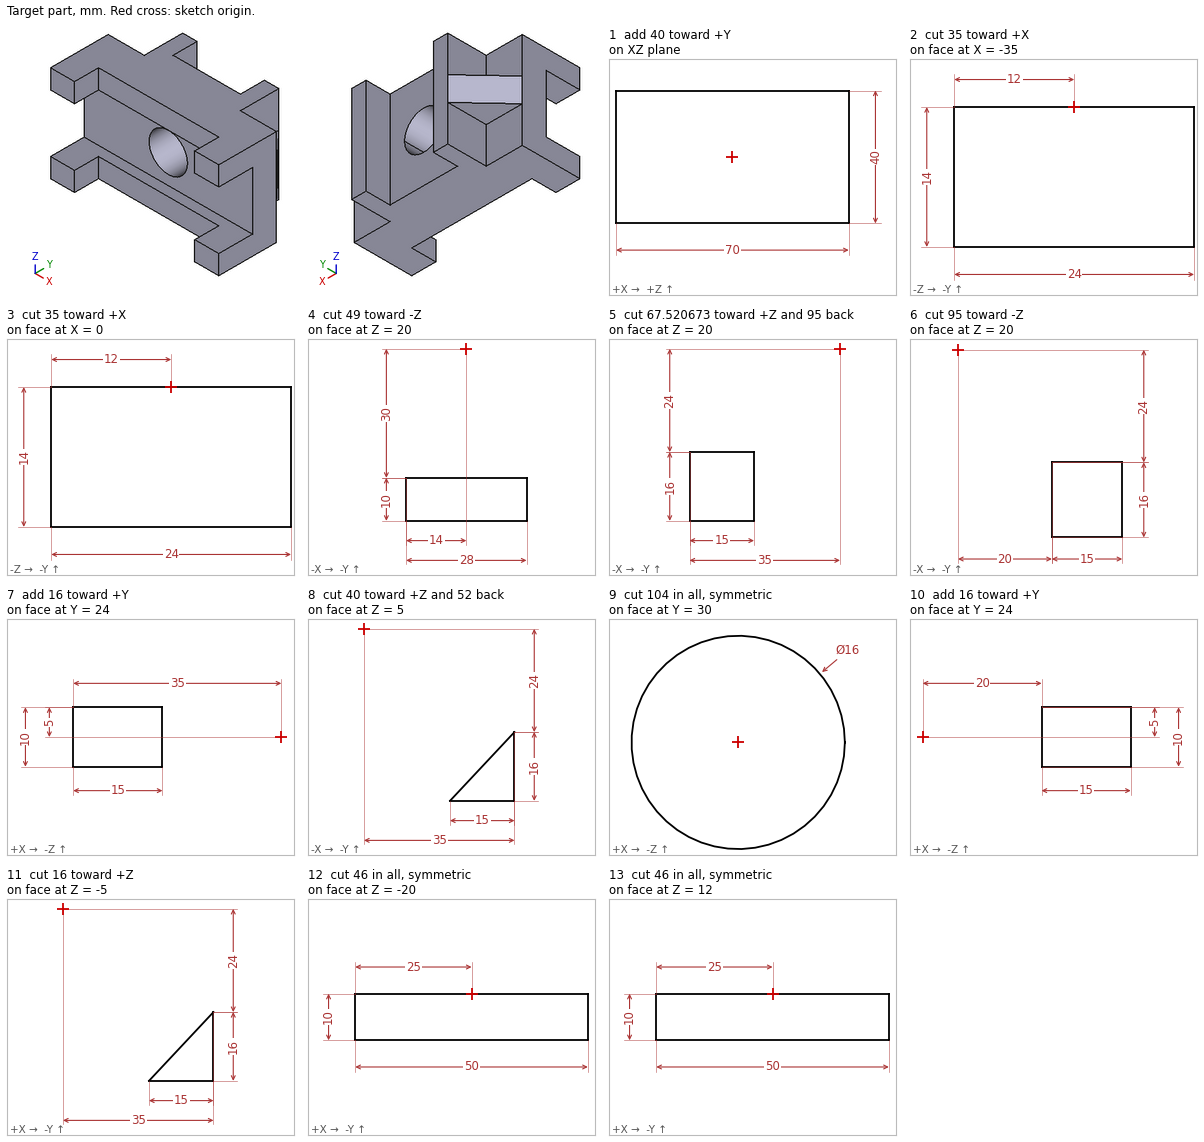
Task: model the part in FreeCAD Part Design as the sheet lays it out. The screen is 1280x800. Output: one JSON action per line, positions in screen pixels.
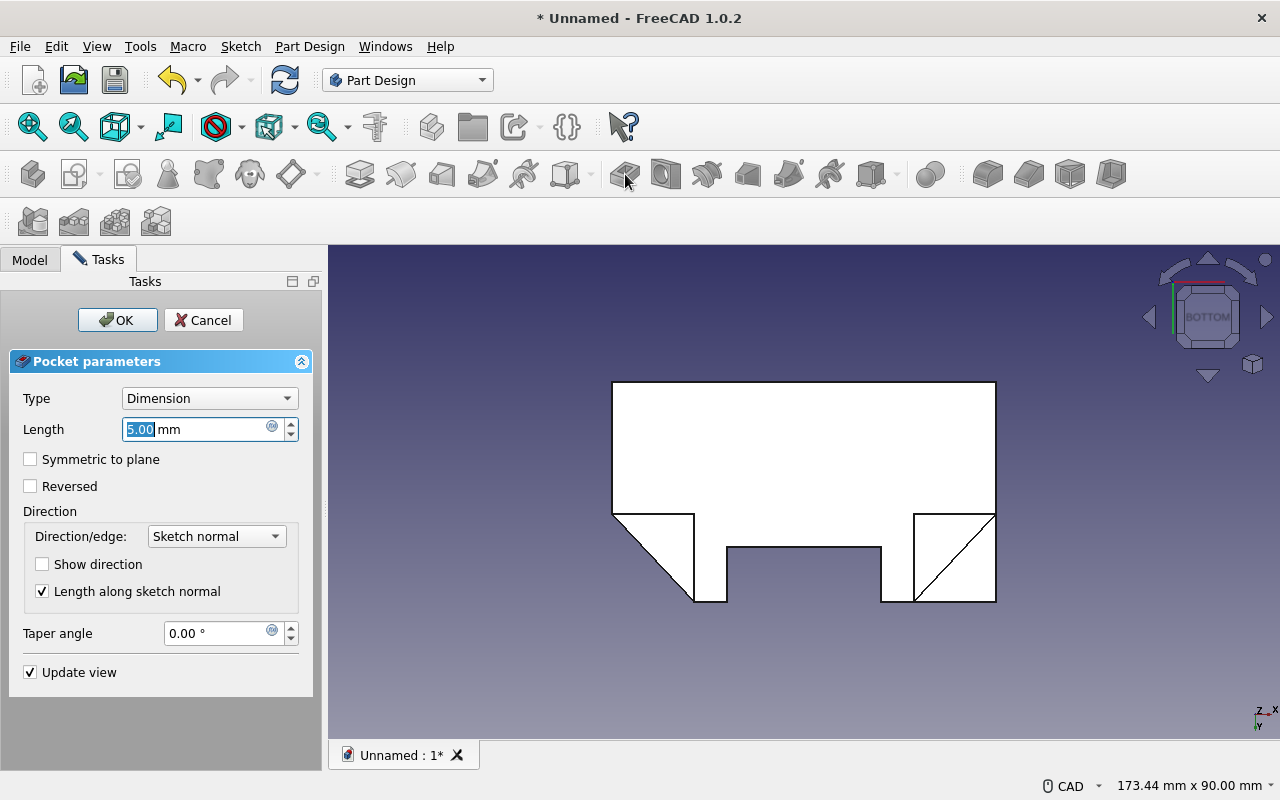
{"action": "type", "text": "16"}
{"action": "key", "text": "Tab"}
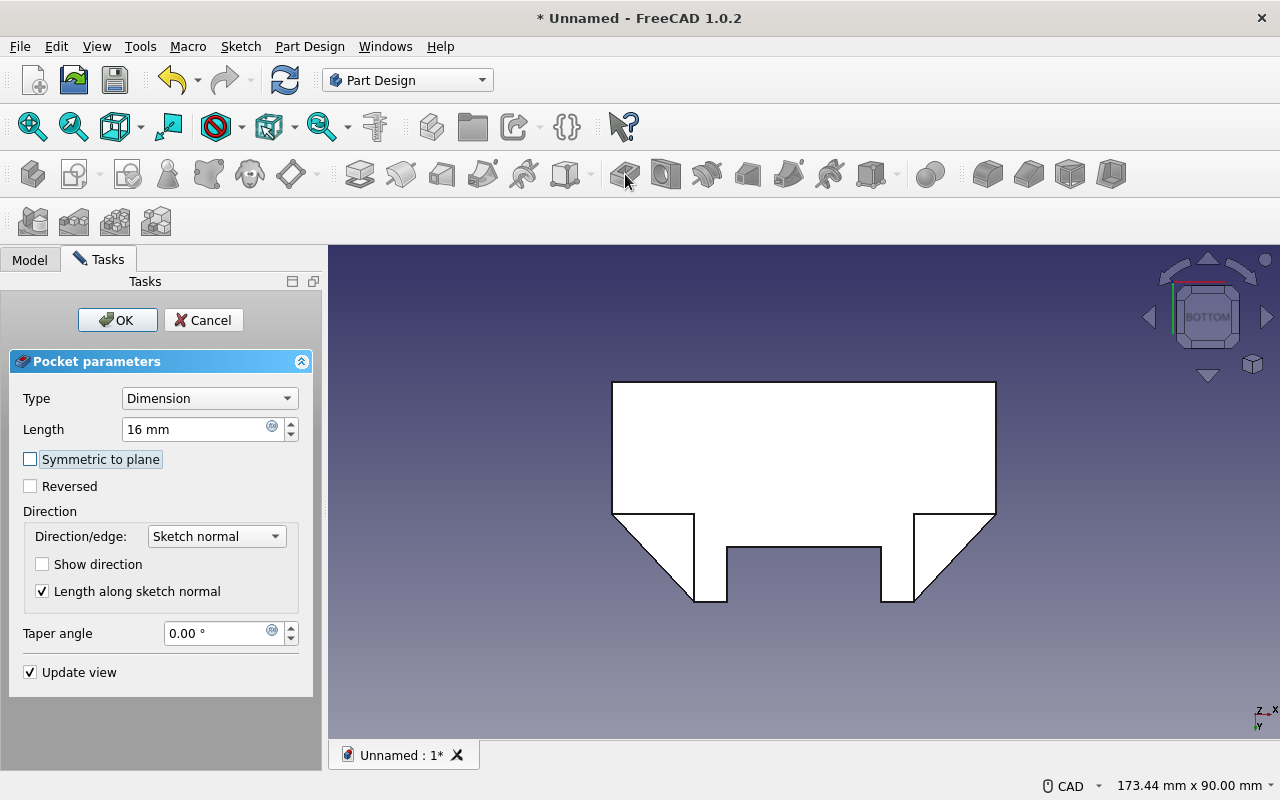
{"action": "left_click", "coordinate": [118, 320]}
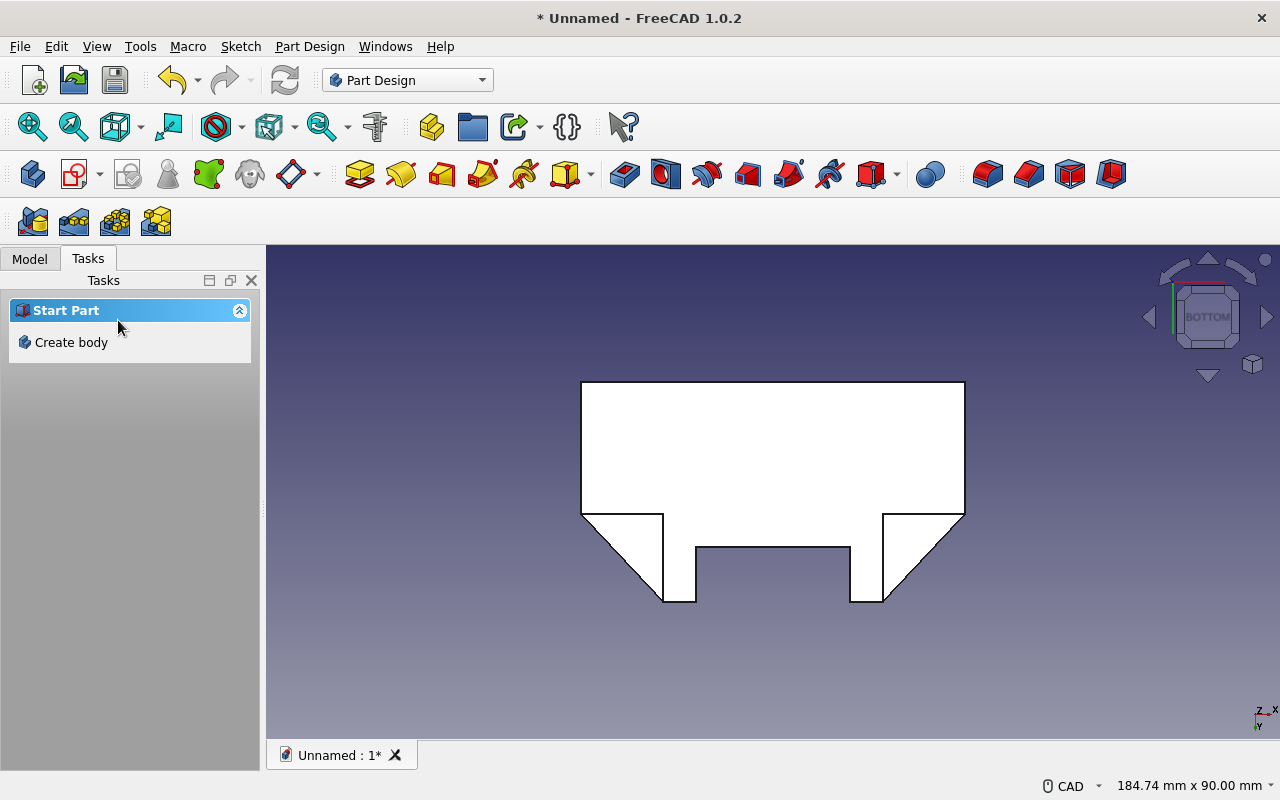
{"action": "key", "text": "v f"}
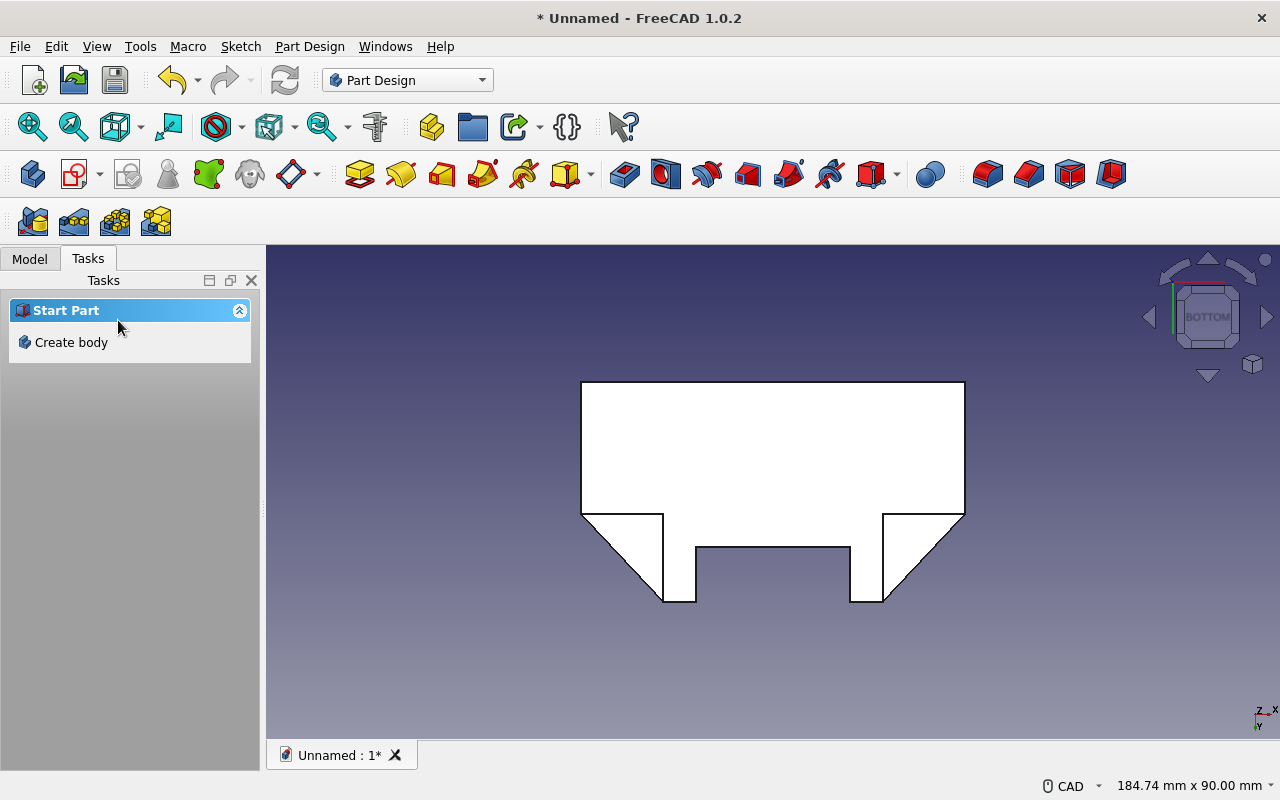
{"action": "left_click", "coordinate": [773, 460]}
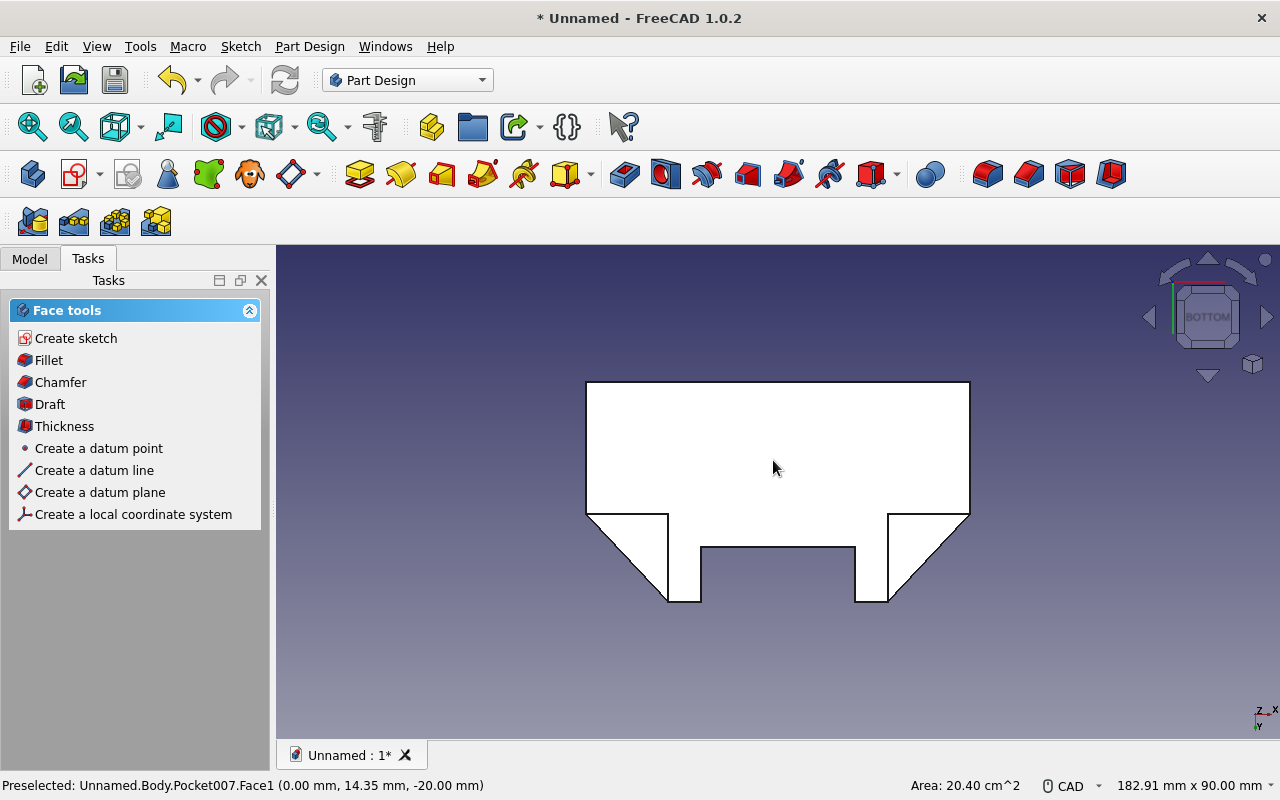
{"action": "left_click", "coordinate": [74, 174]}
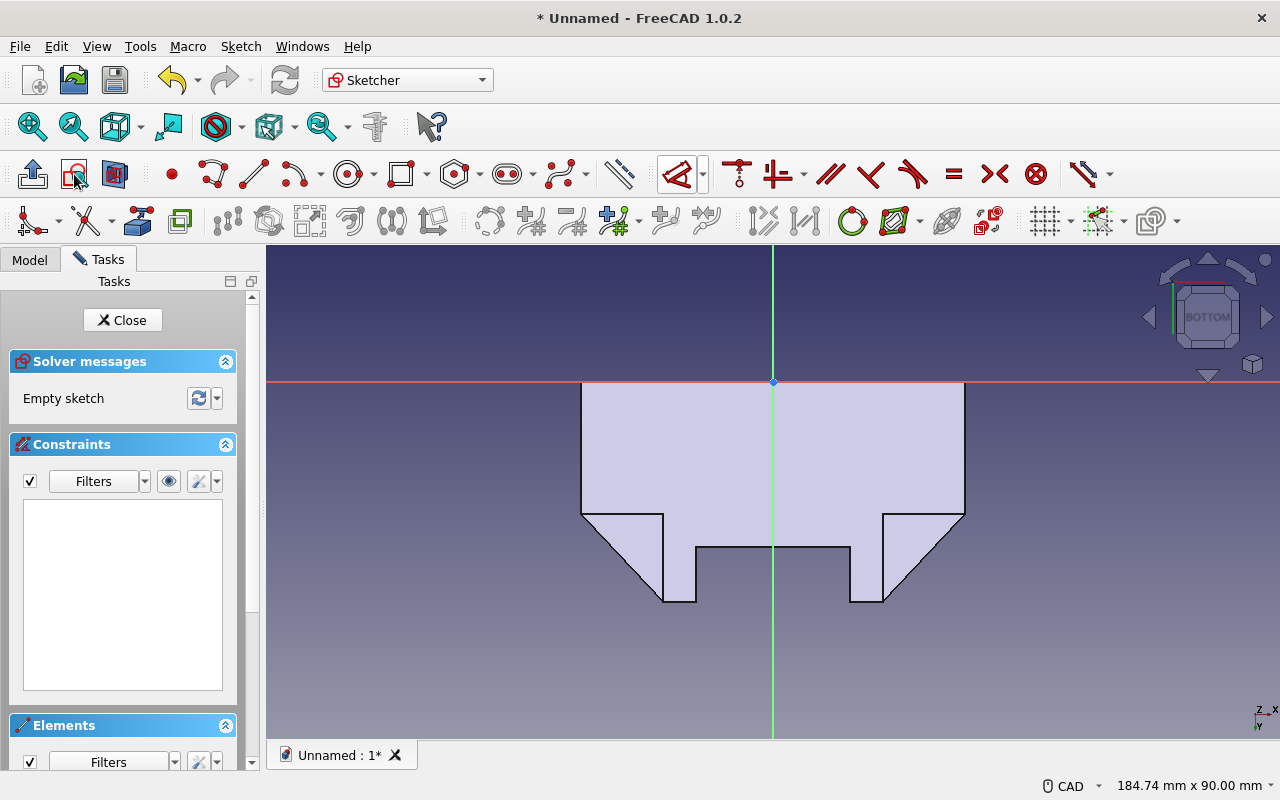
{"action": "scroll", "coordinate": [829, 342], "scroll_direction": "up", "scroll_amount": 4}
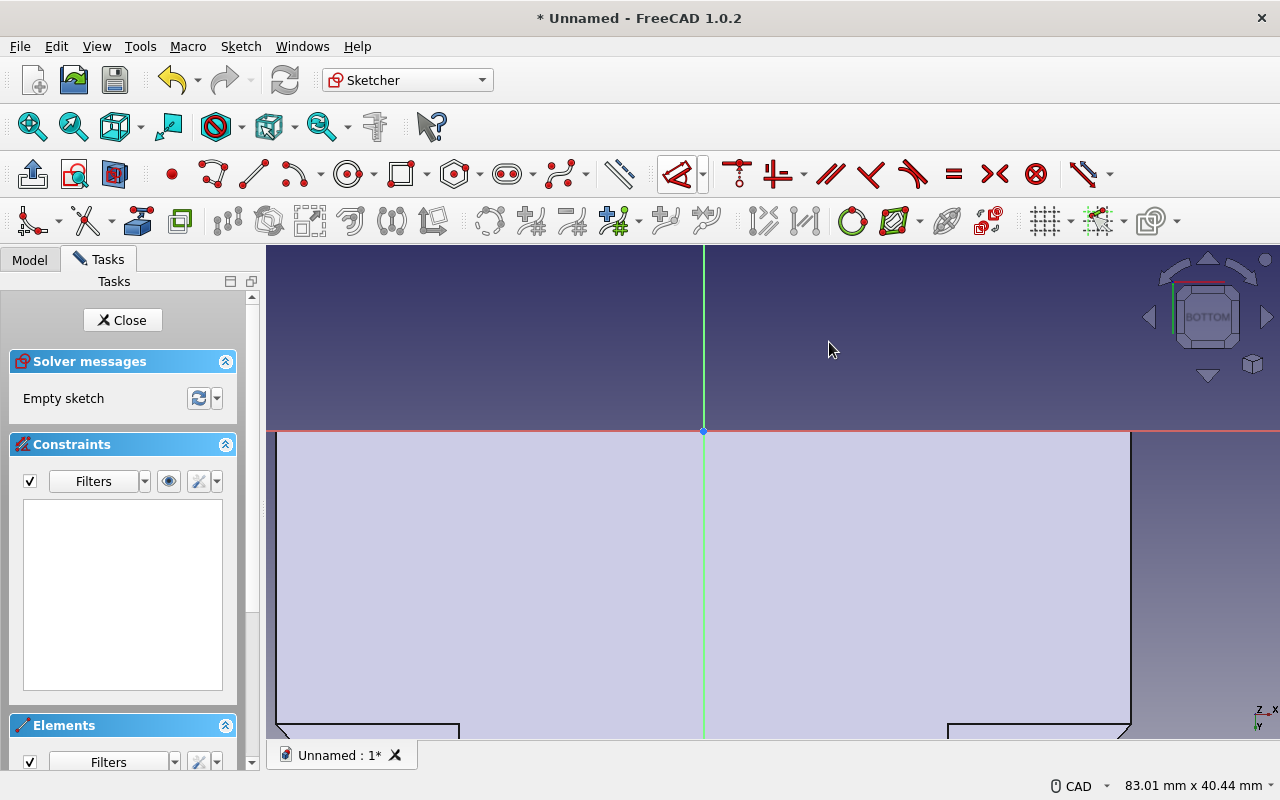
{"action": "key", "text": "g r"}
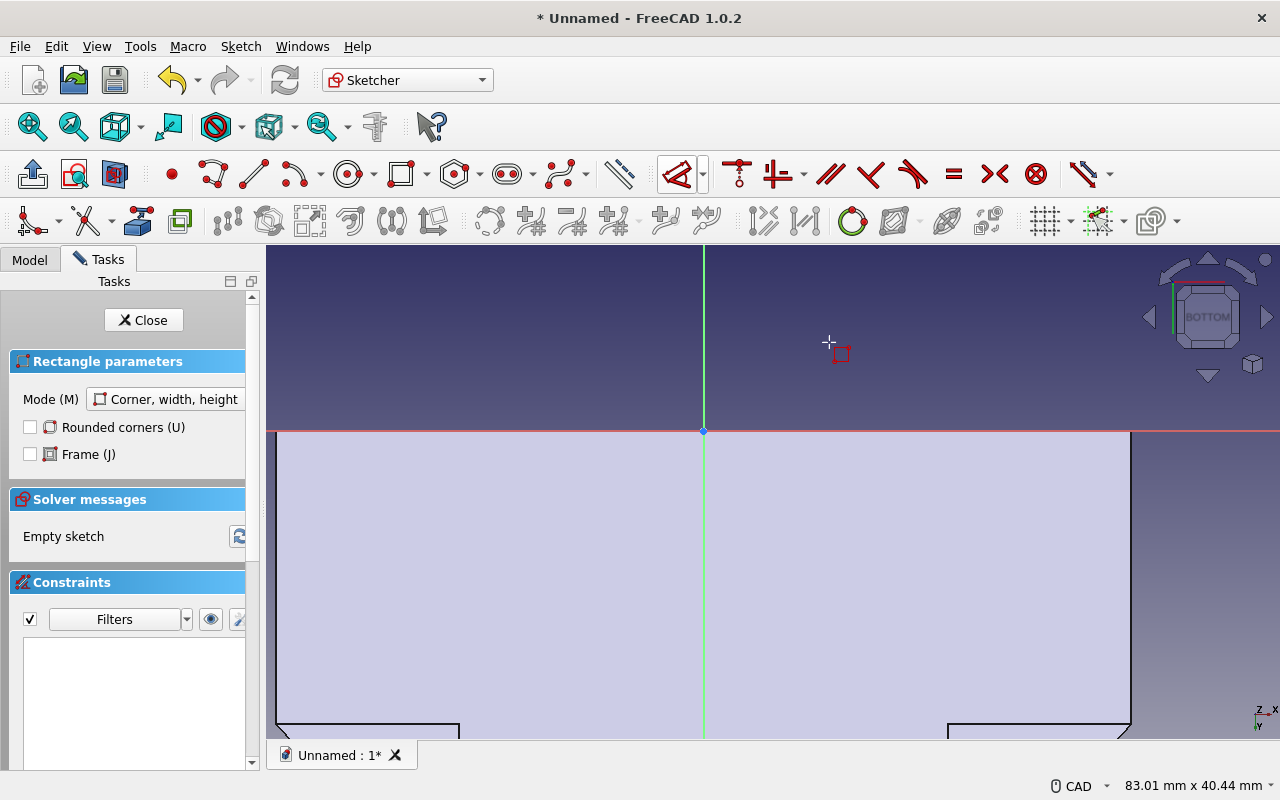
{"action": "left_click", "coordinate": [398, 431]}
{"action": "left_click", "coordinate": [1009, 553]}
{"action": "key", "text": "Escape"}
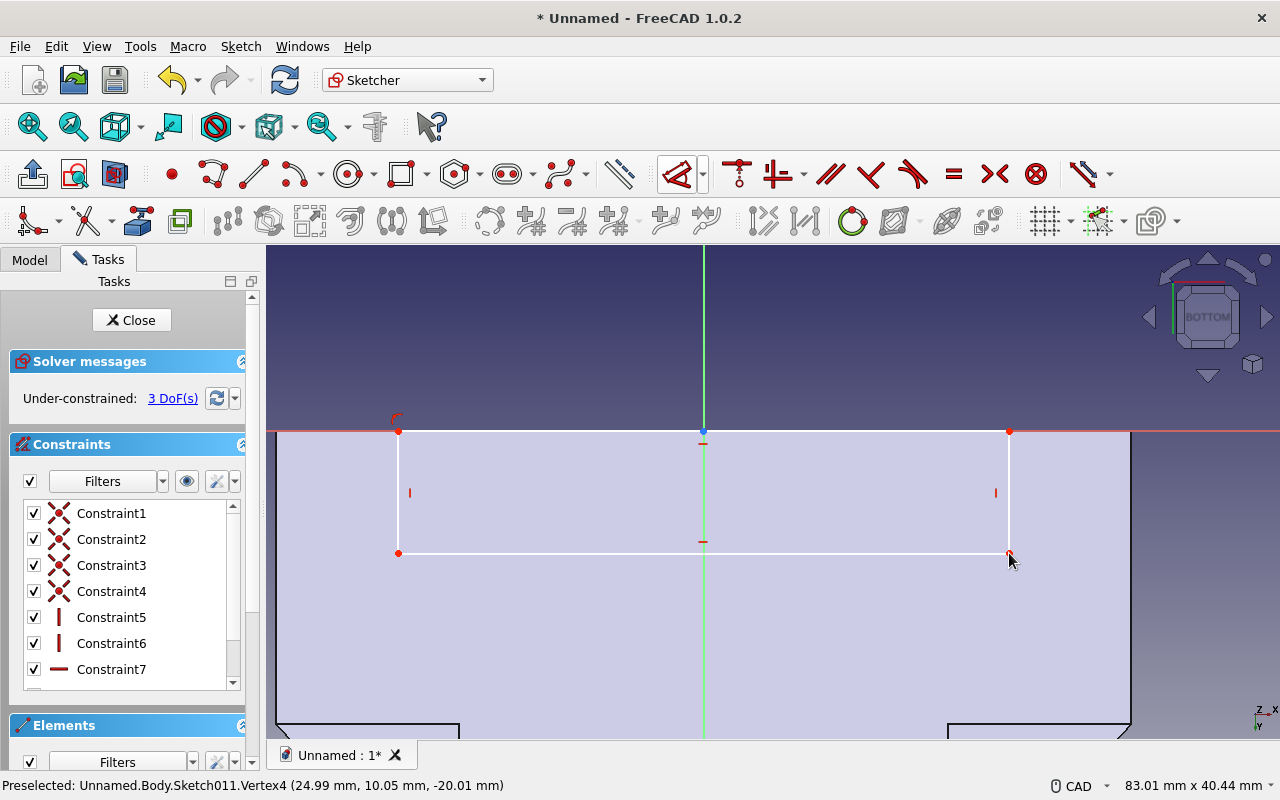
{"action": "left_click", "coordinate": [398, 468]}